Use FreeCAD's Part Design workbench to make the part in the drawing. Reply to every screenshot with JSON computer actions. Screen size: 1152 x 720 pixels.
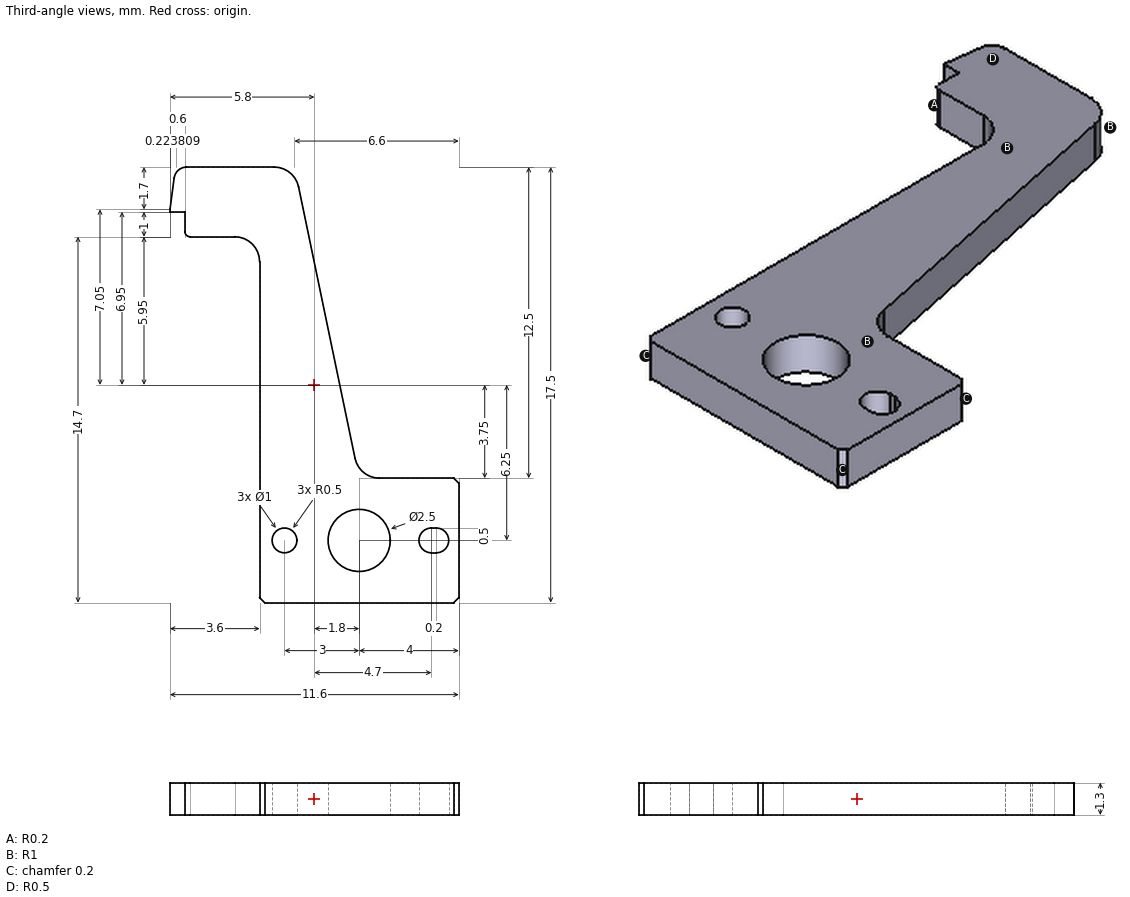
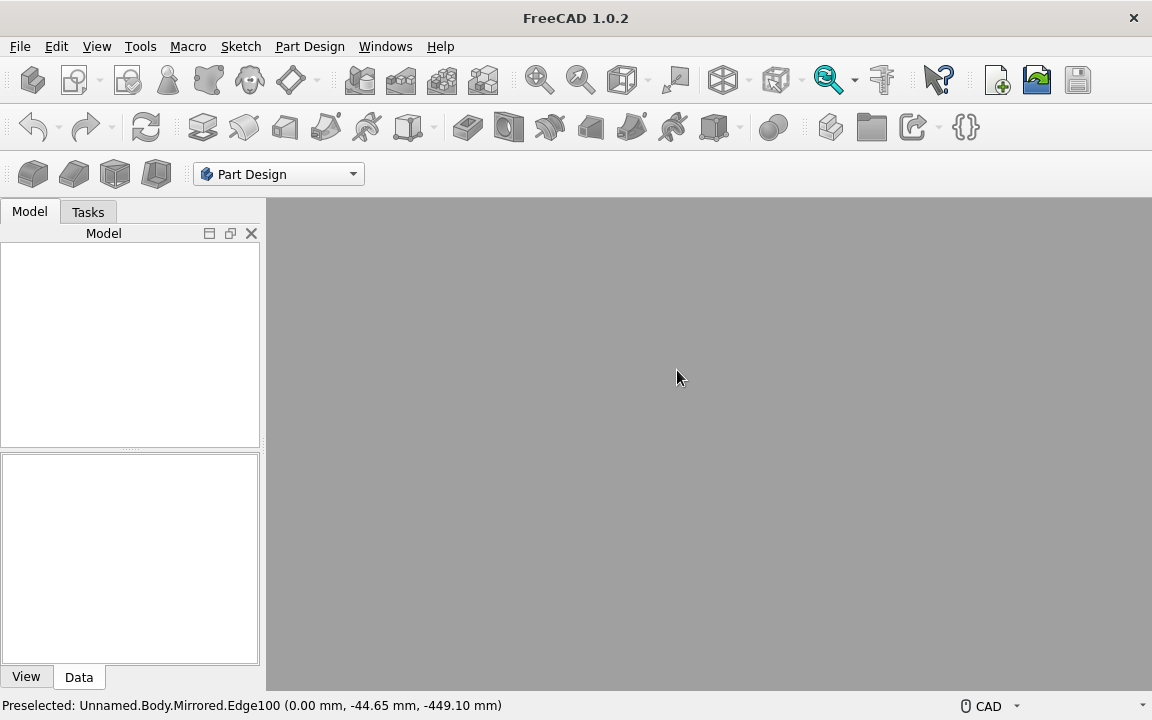
{"action": "key", "text": "ctrl+n"}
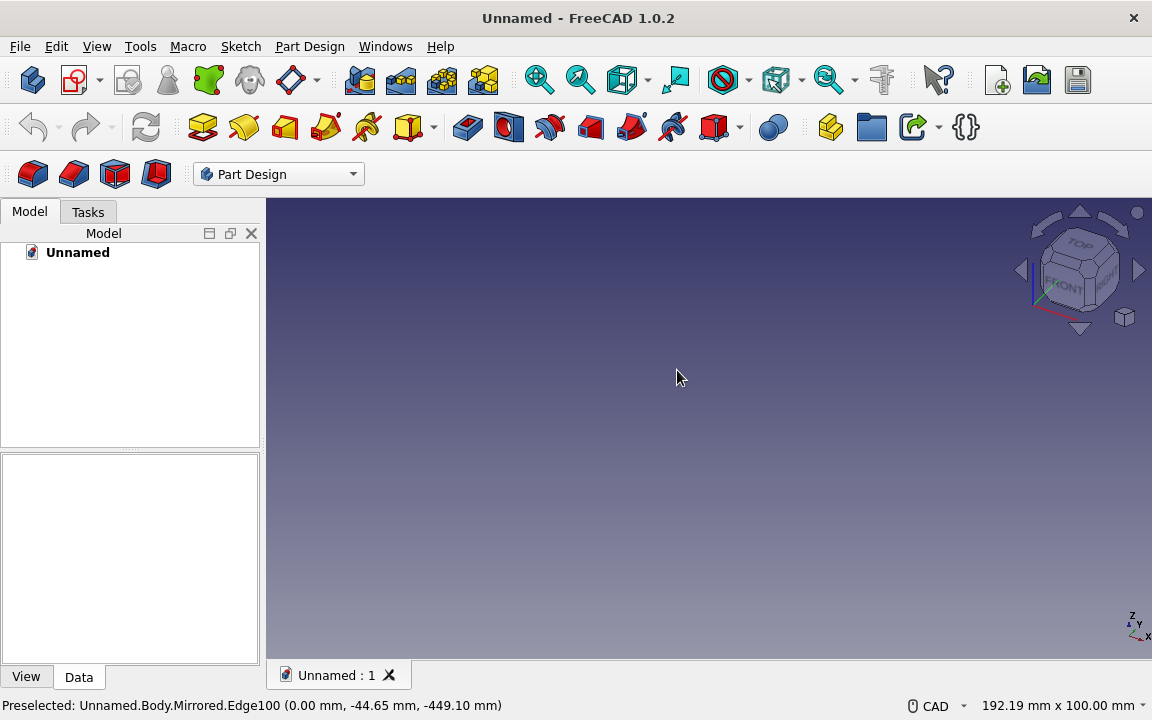
{"action": "left_click", "coordinate": [74, 80]}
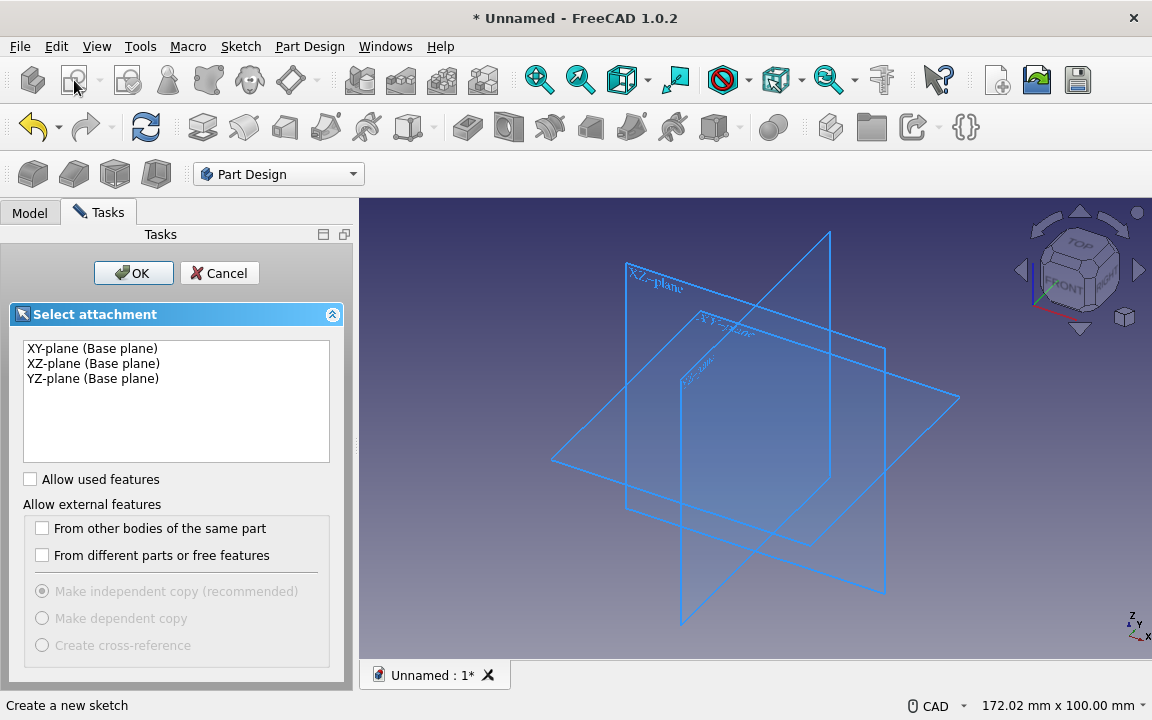
{"action": "left_click", "coordinate": [84, 348]}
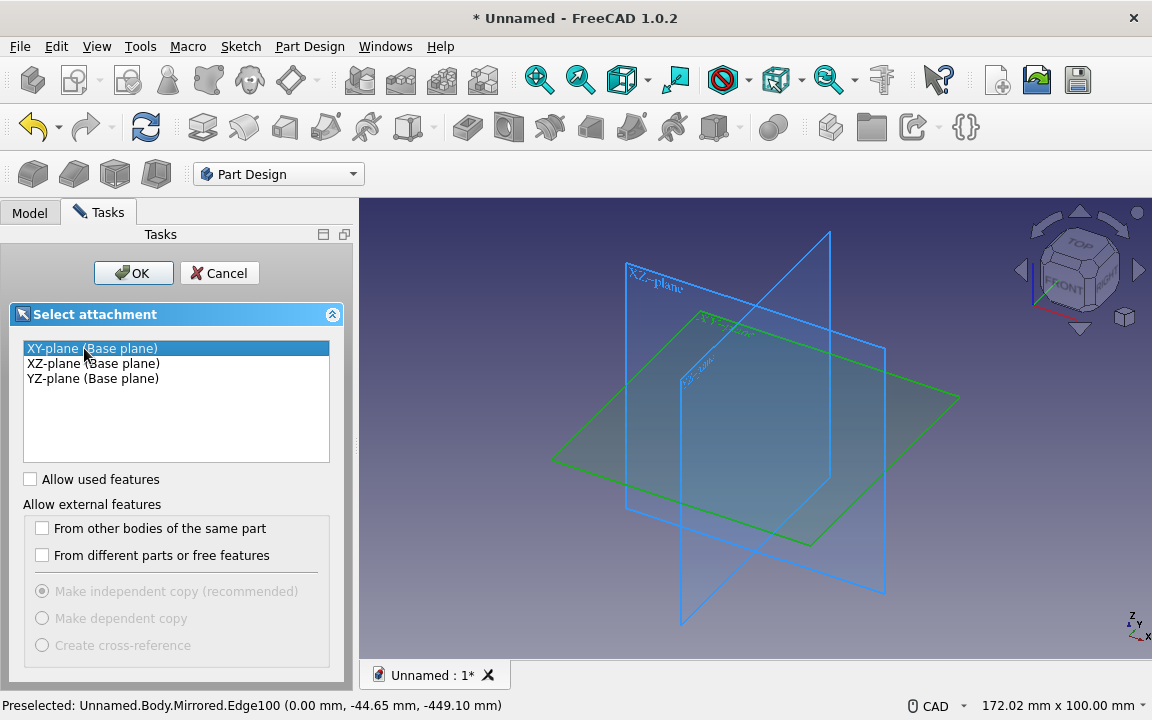
{"action": "left_click", "coordinate": [134, 273]}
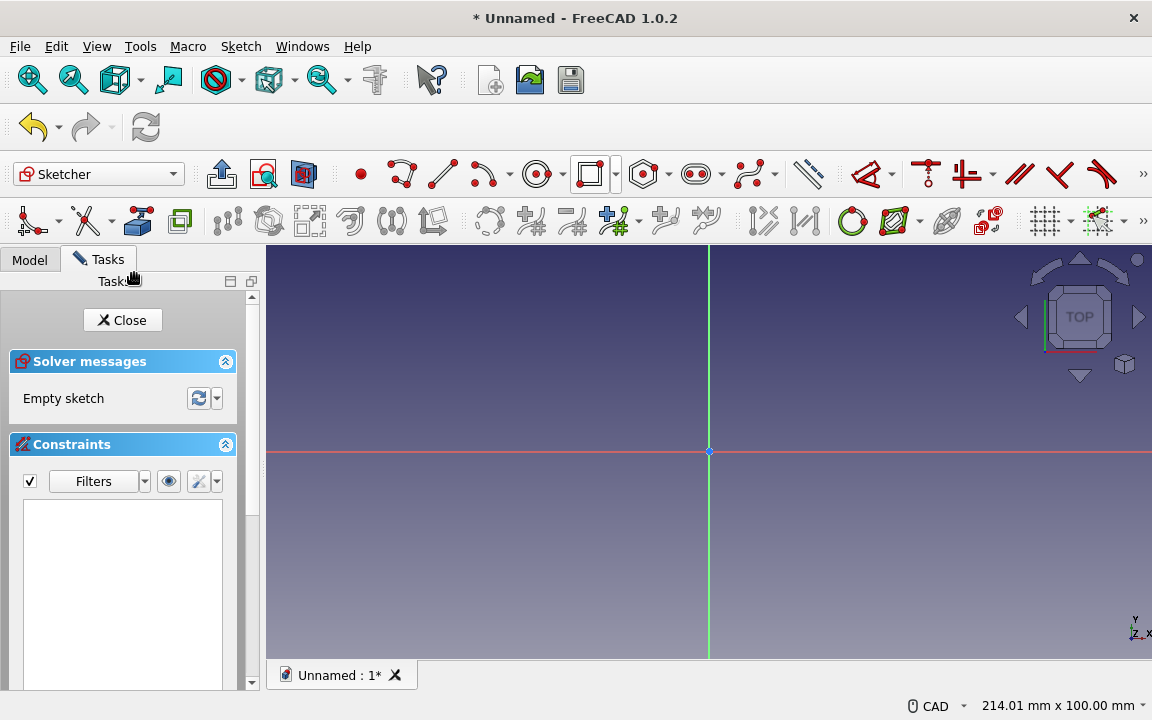
{"action": "scroll", "coordinate": [739, 452], "scroll_direction": "up", "scroll_amount": 6}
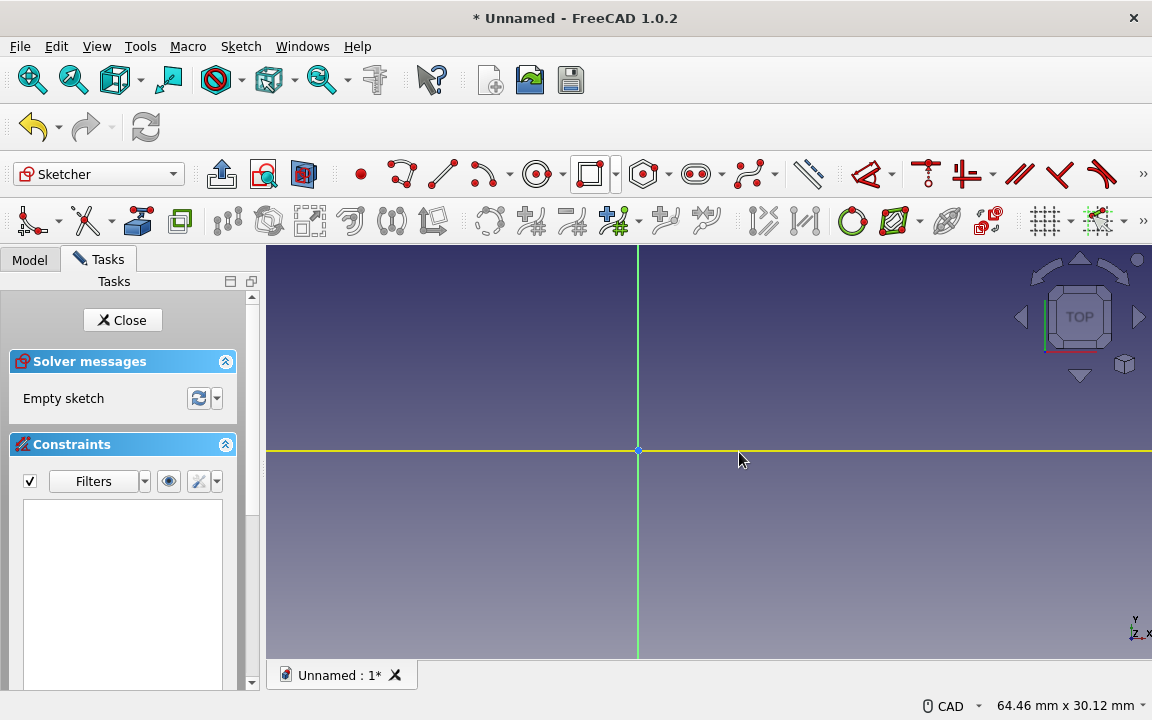
{"action": "key", "text": "g v"}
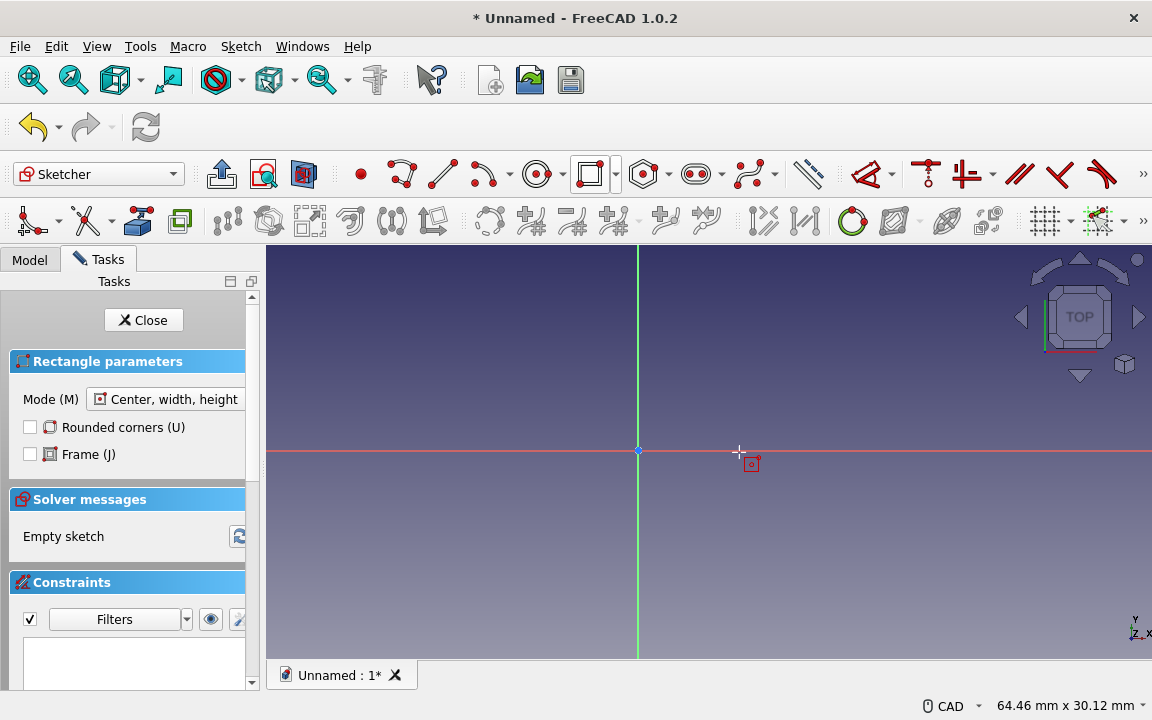
{"action": "left_click", "coordinate": [638, 451]}
{"action": "left_click", "coordinate": [718, 331]}
{"action": "key", "text": "Escape"}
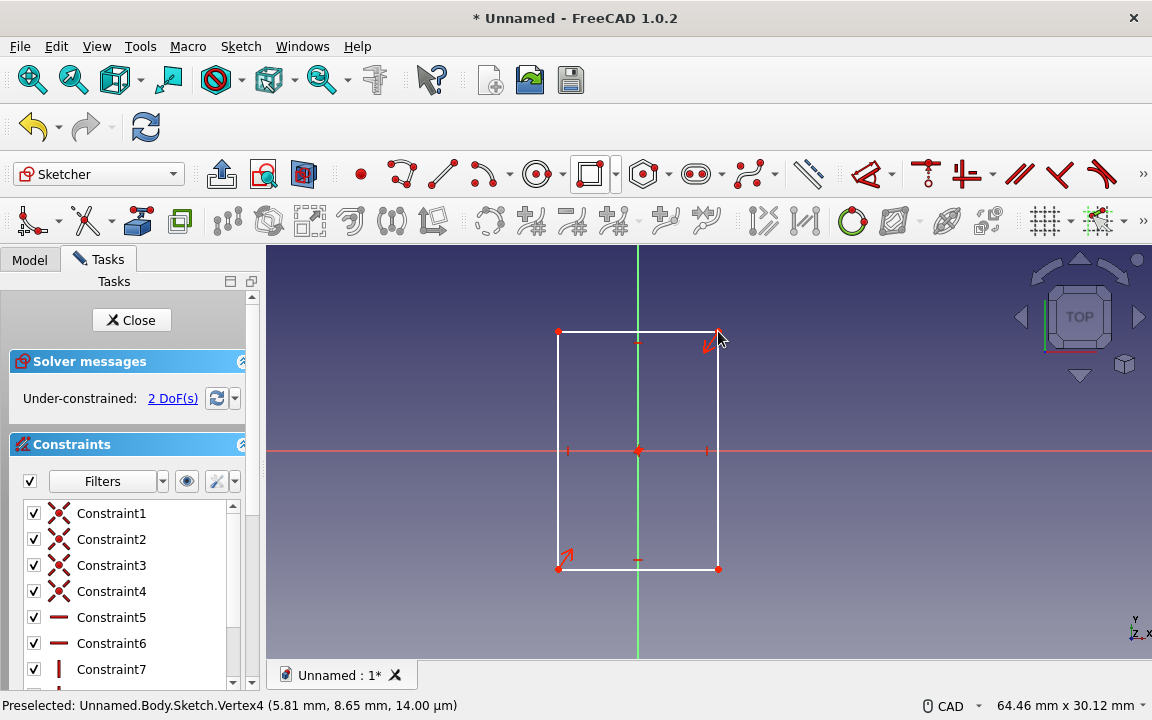
{"action": "left_click", "coordinate": [866, 174]}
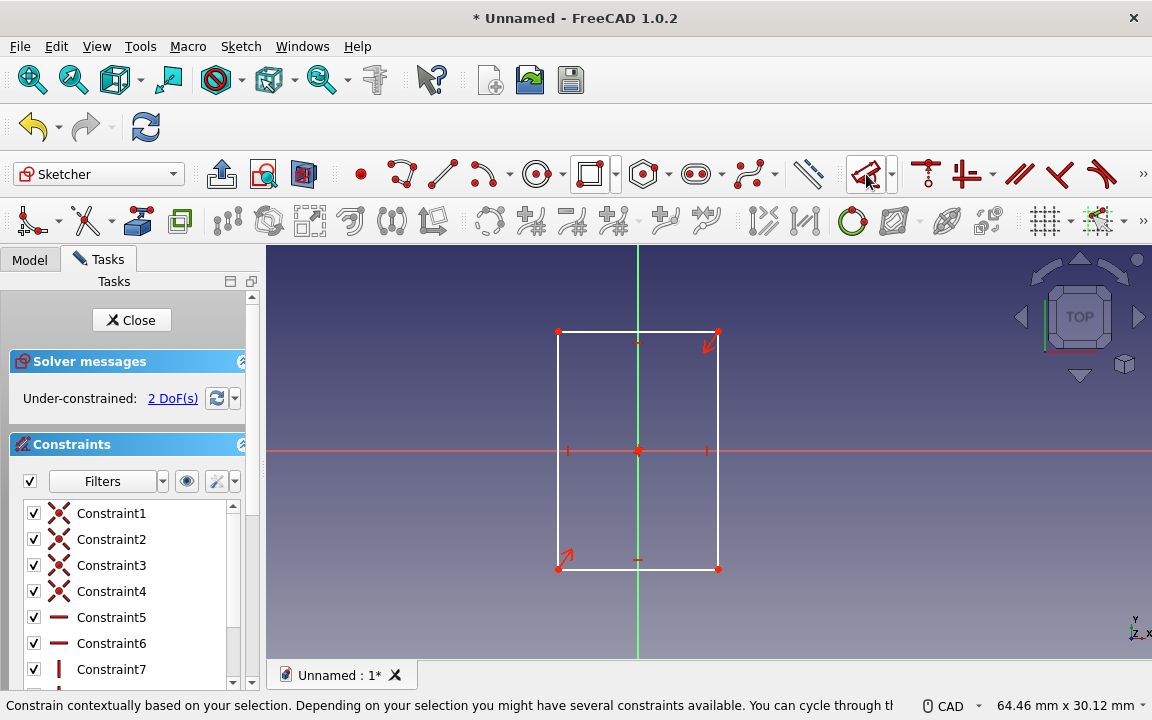
{"action": "left_click", "coordinate": [606, 570]}
{"action": "left_click", "coordinate": [601, 604]}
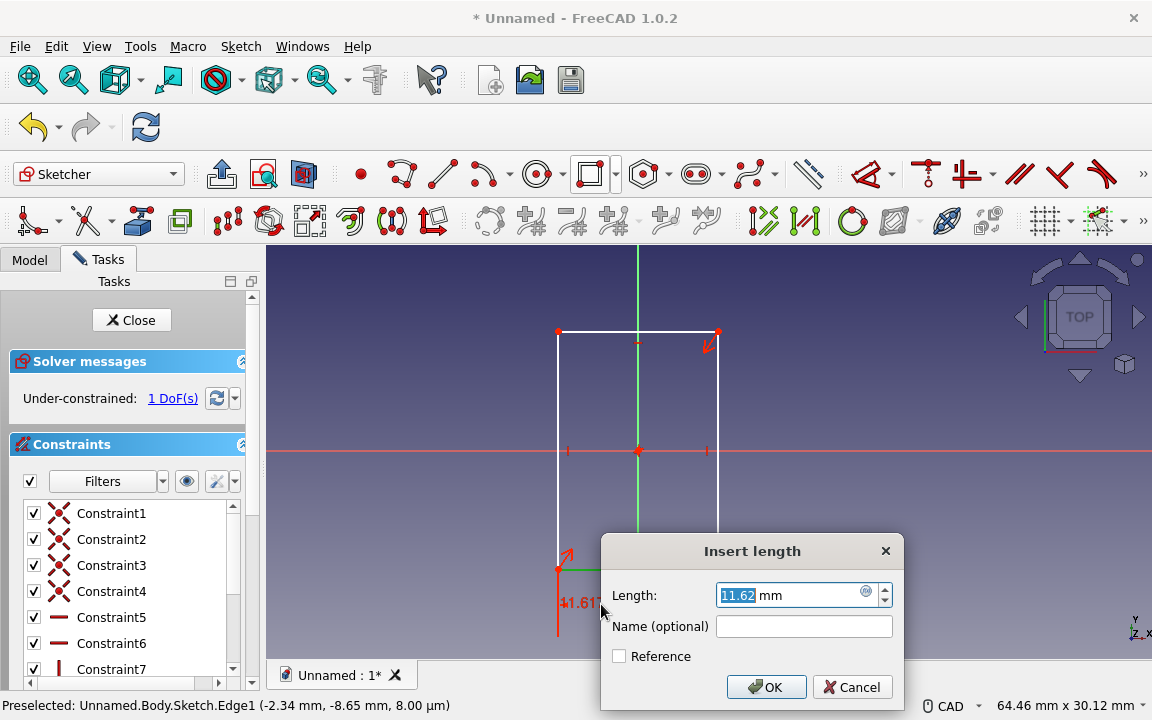
{"action": "type", "text": "11.6"}
{"action": "key", "text": "Return"}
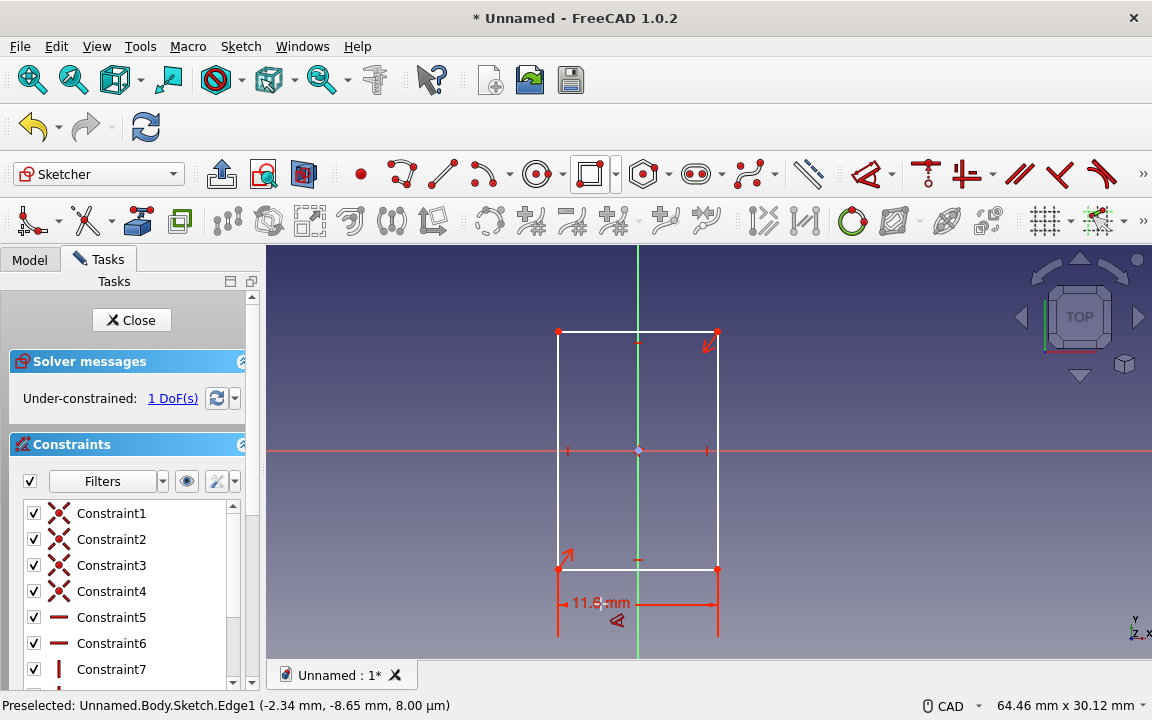
{"action": "left_click", "coordinate": [718, 498]}
{"action": "left_click", "coordinate": [752, 396]}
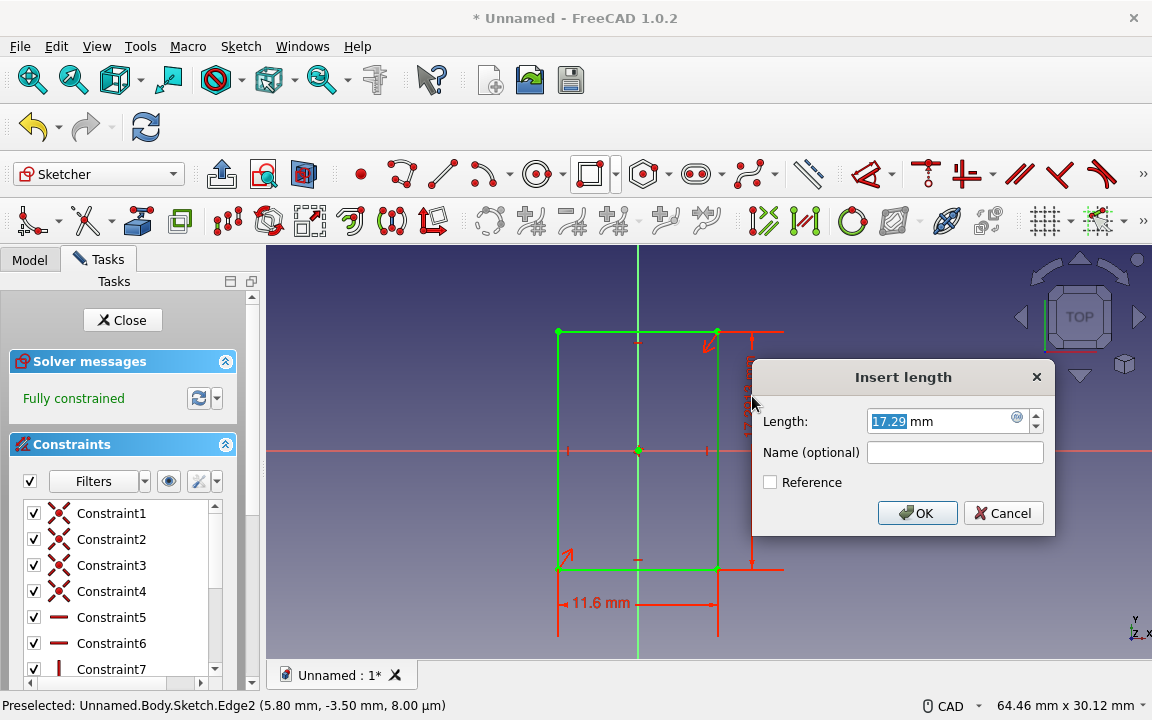
{"action": "type", "text": "17.5"}
{"action": "key", "text": "Return"}
{"action": "key", "text": "Escape"}